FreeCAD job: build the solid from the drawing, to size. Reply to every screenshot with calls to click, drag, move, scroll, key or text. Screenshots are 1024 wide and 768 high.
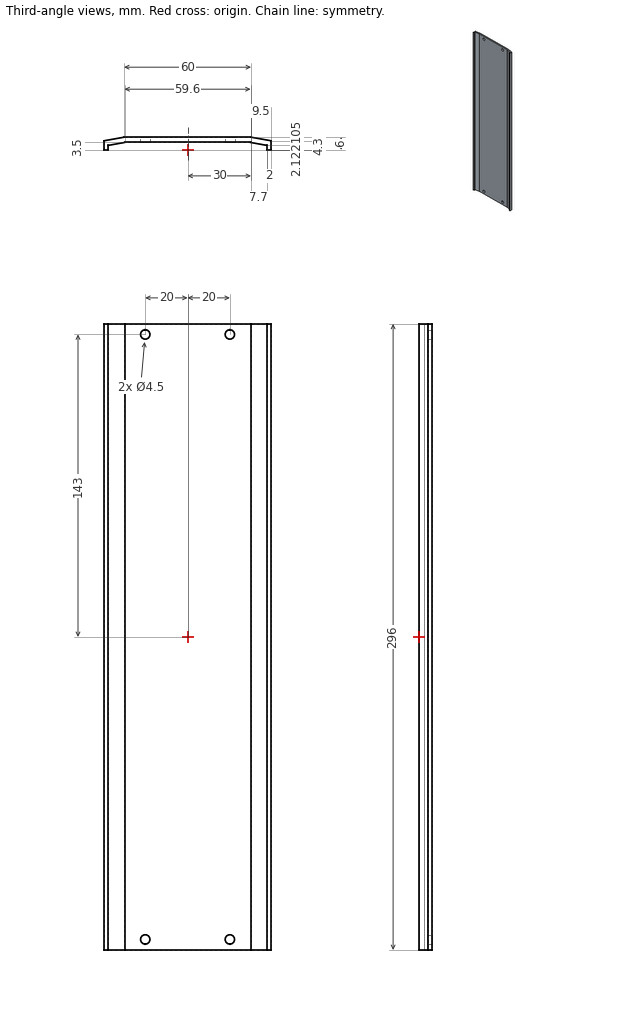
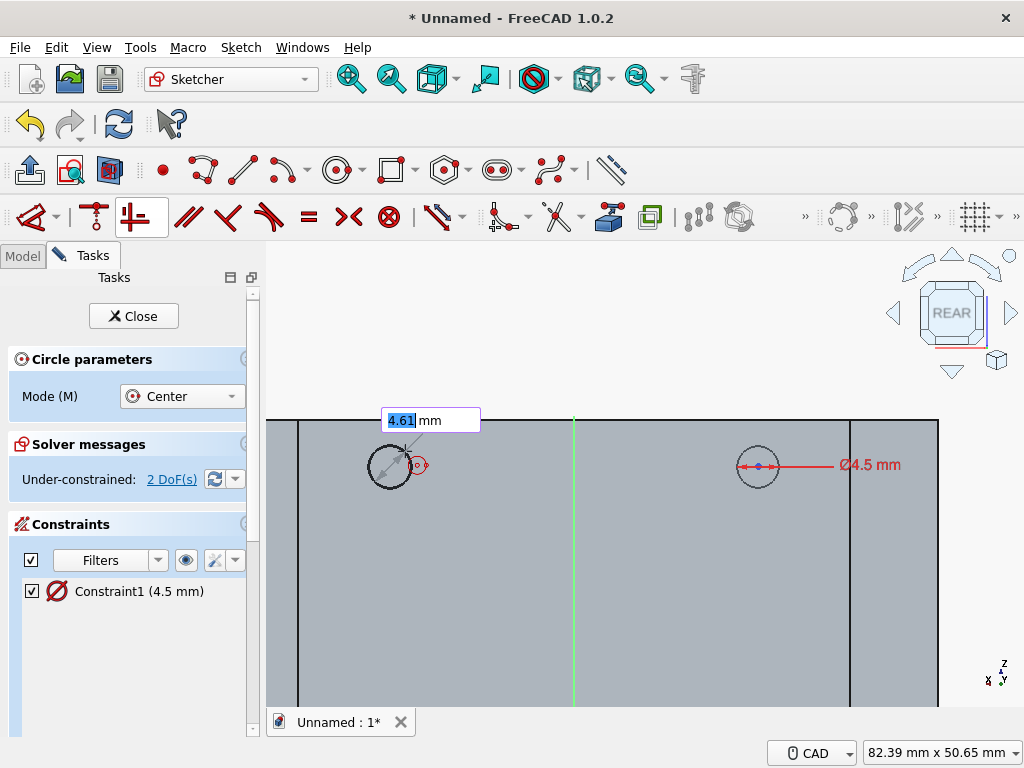
text(4.5)
key(Return)
key(Escape)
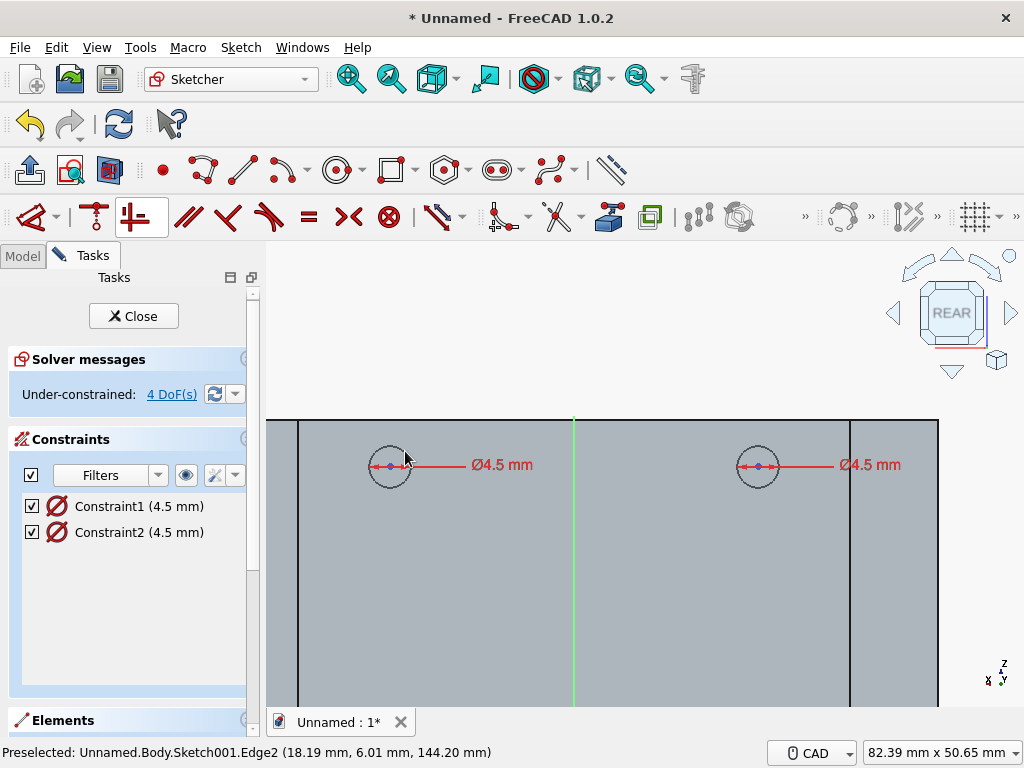
click(758, 467)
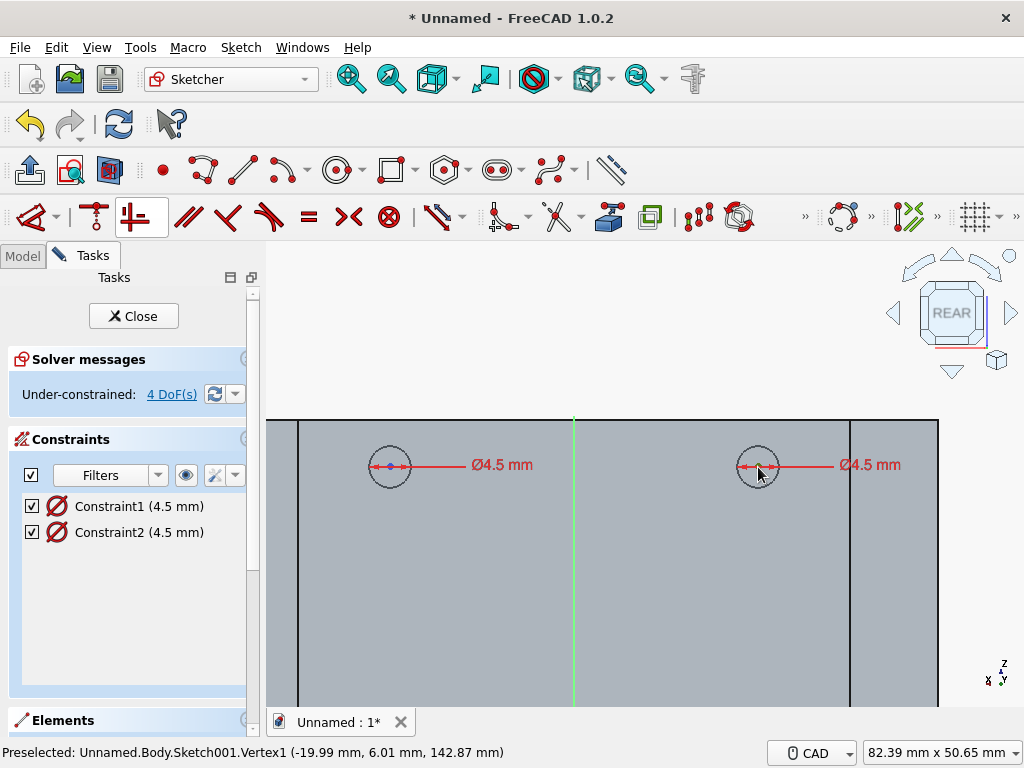
click(390, 467)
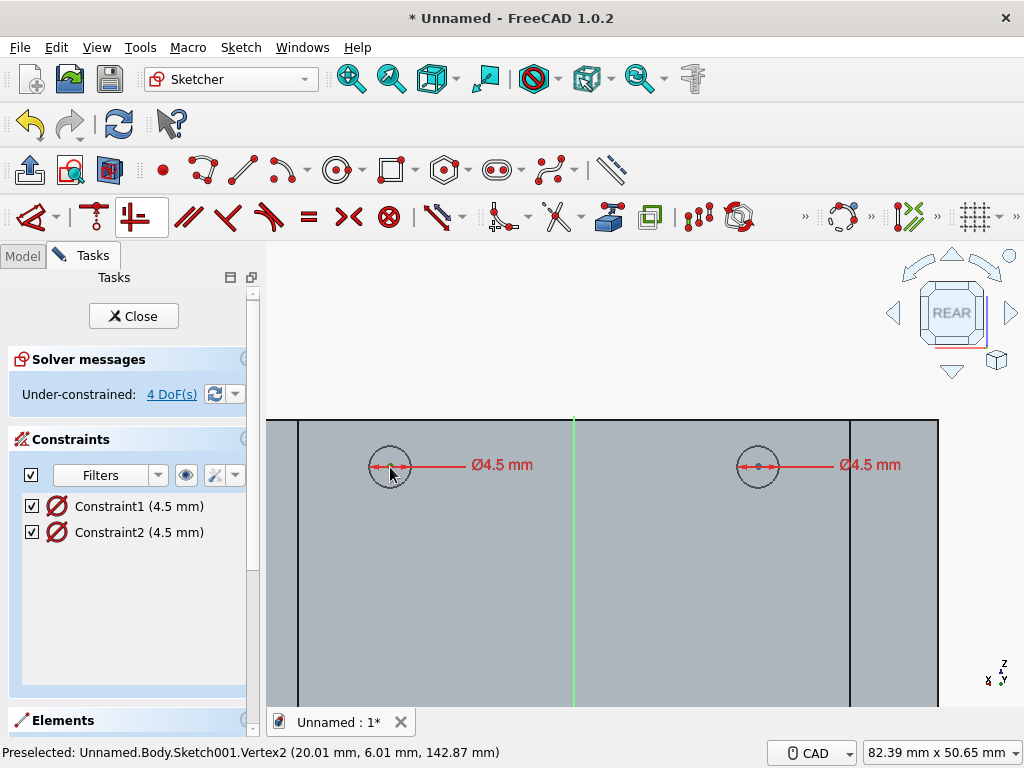
key(h)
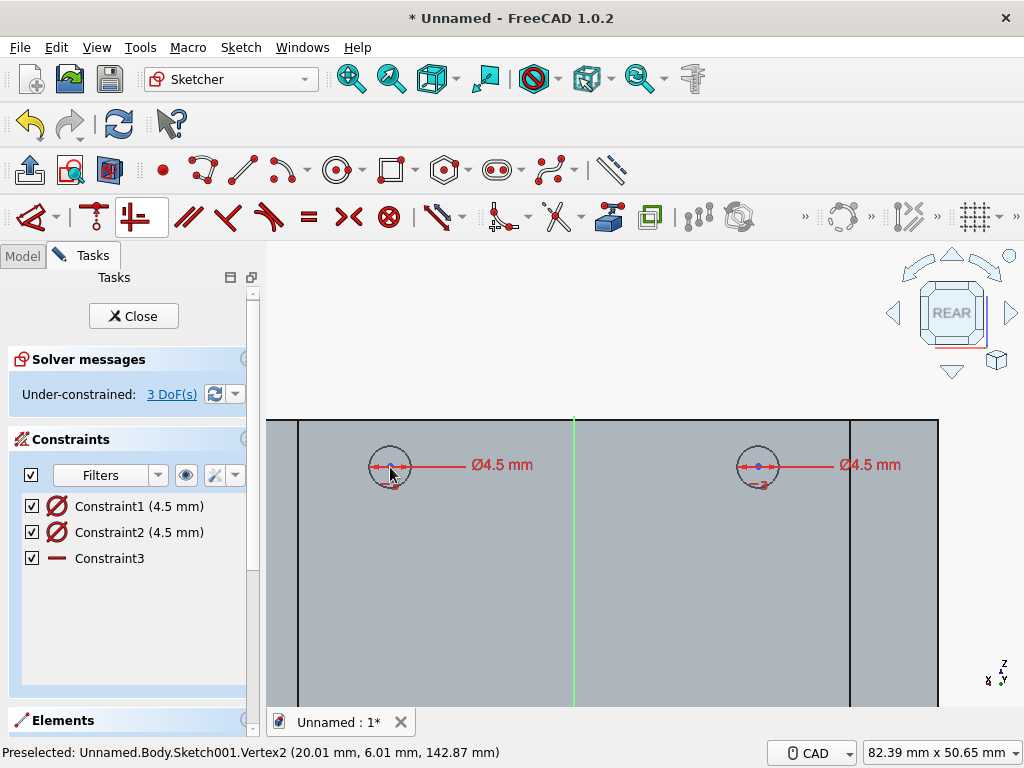
key(d)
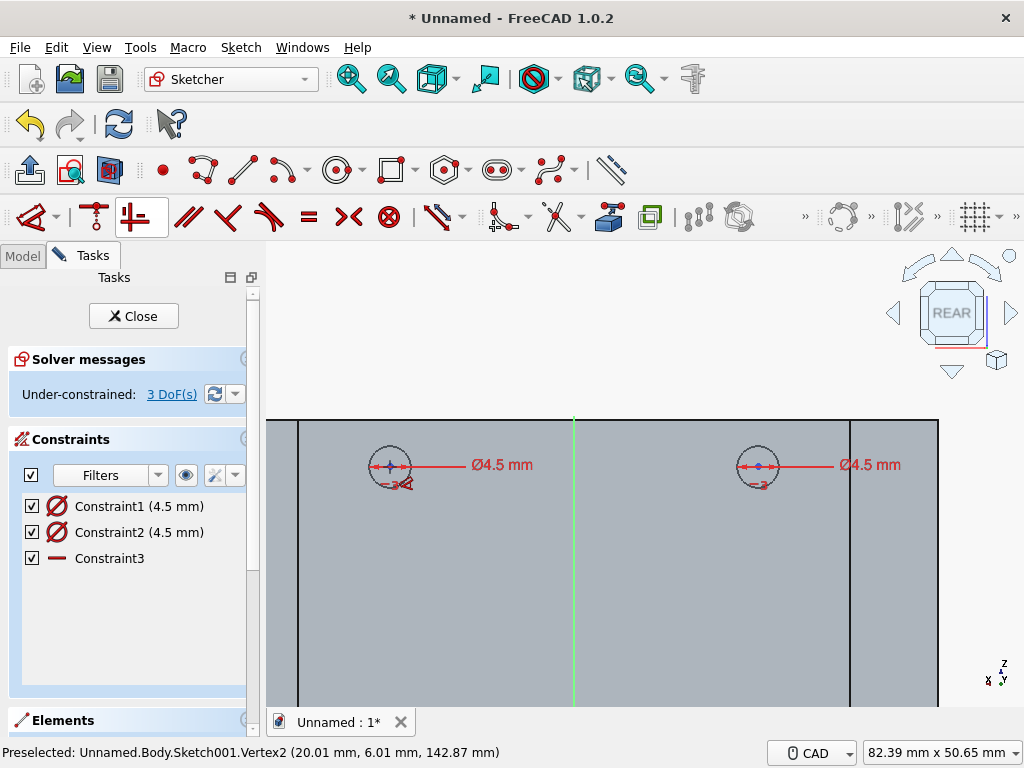
click(758, 467)
click(666, 433)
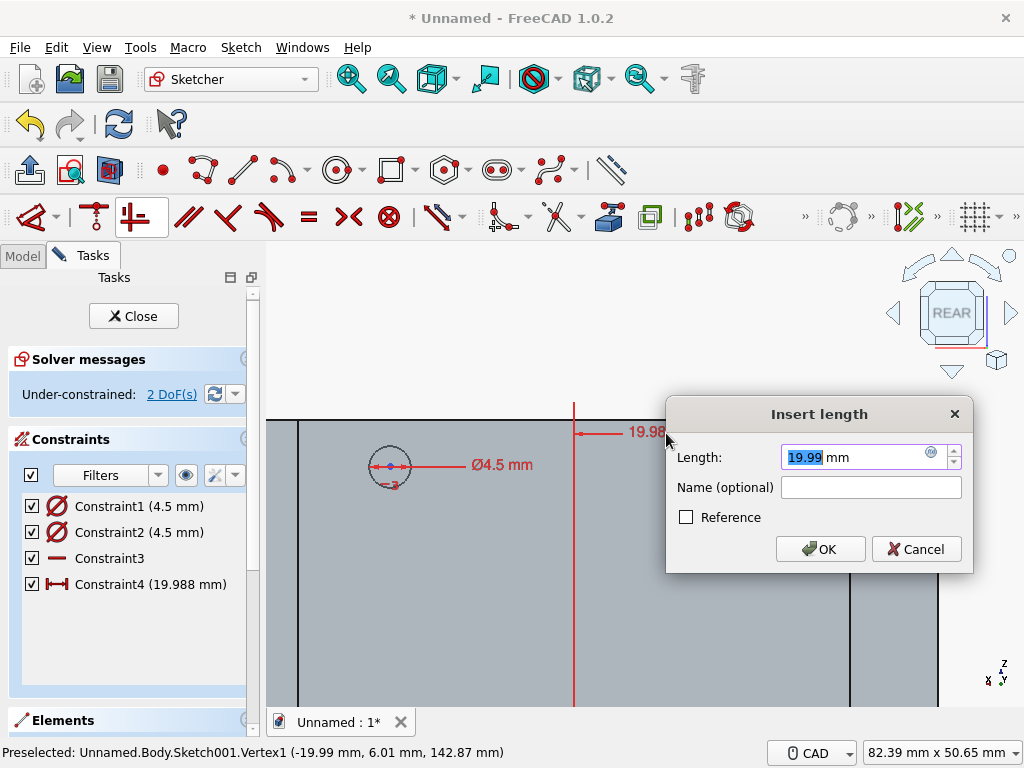
text(20)
key(Return)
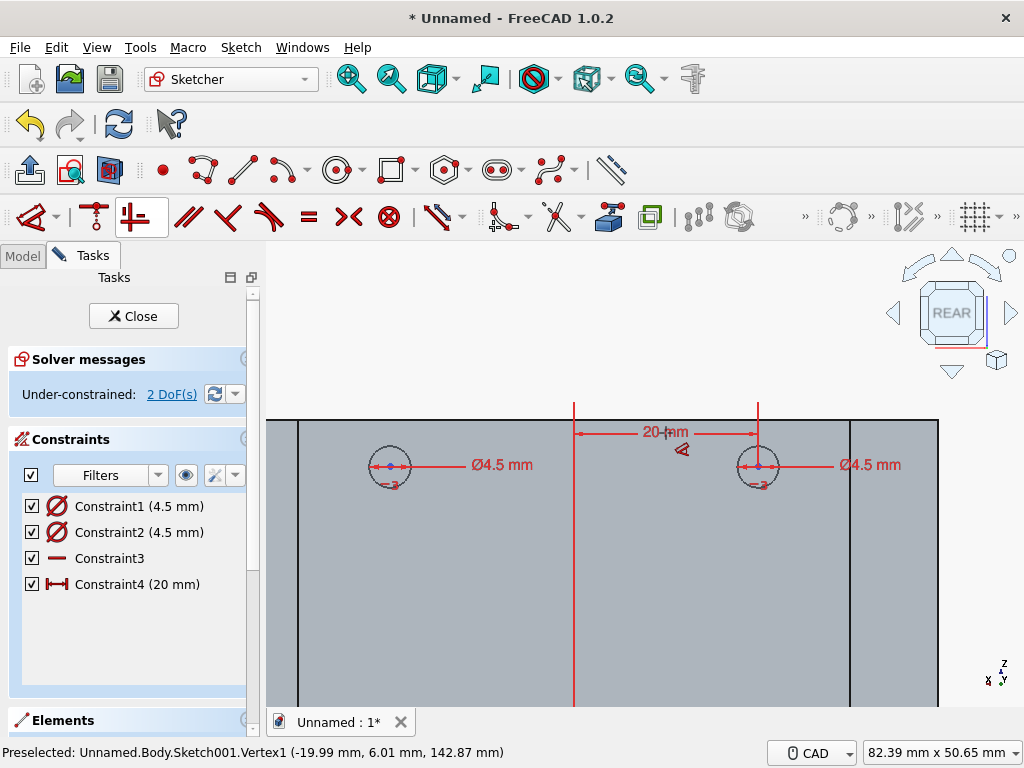
click(390, 467)
click(482, 433)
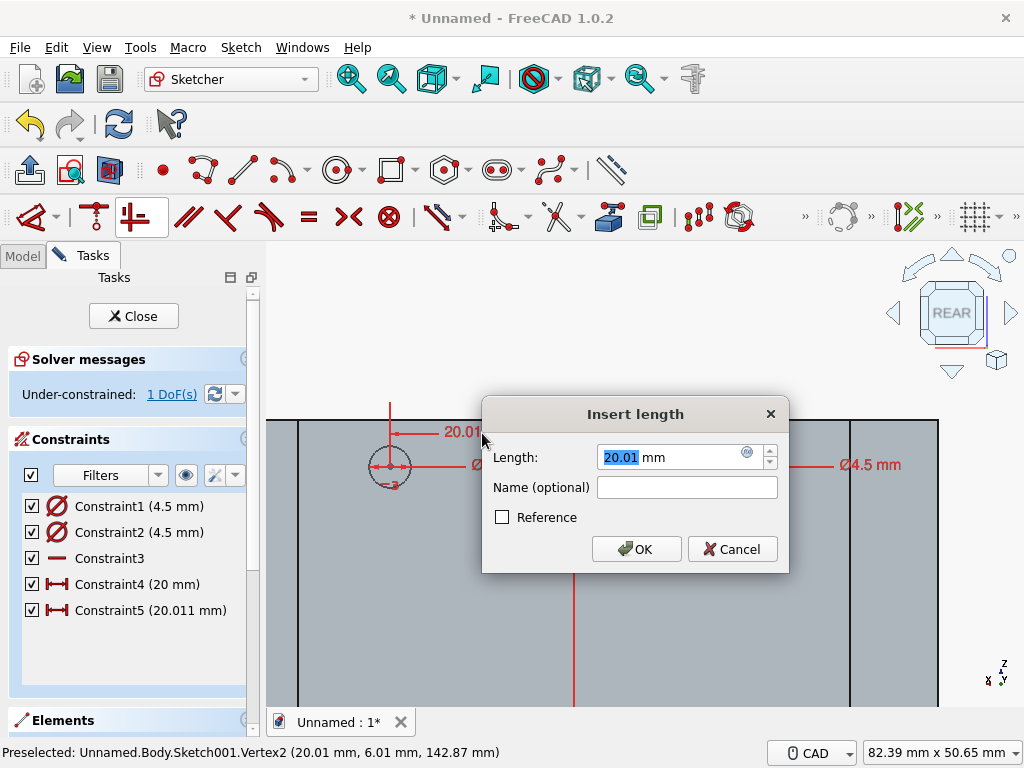
text(20)
key(Return)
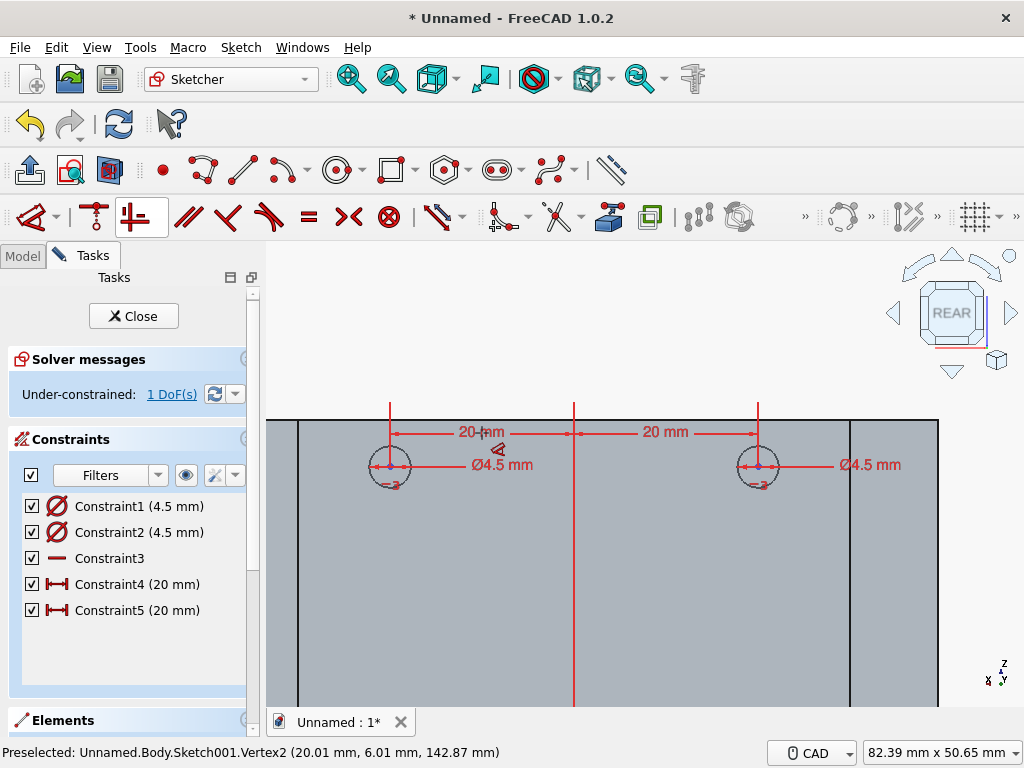
click(758, 467)
click(792, 573)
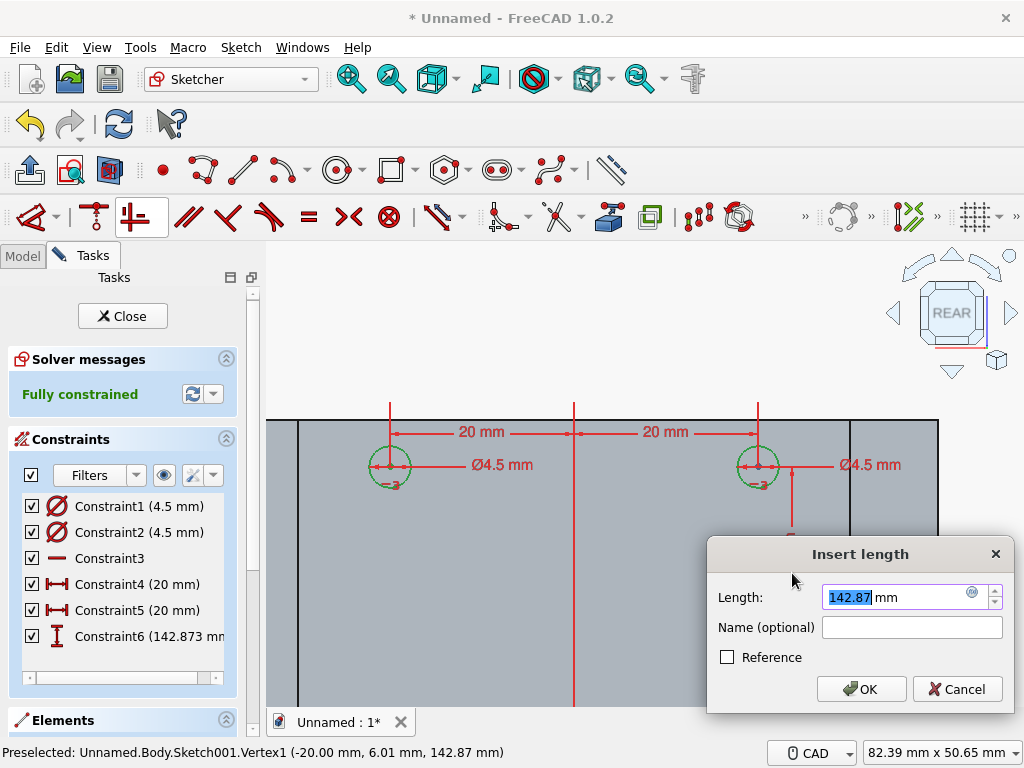
text(143)
key(Return)
key(Escape)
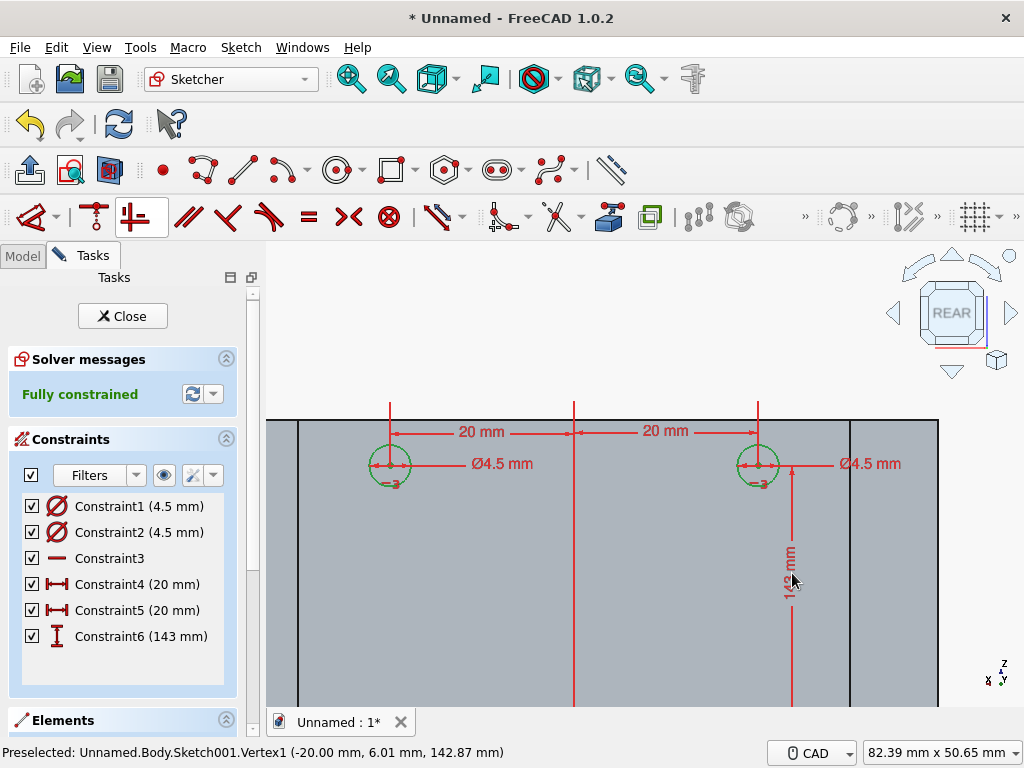
click(123, 316)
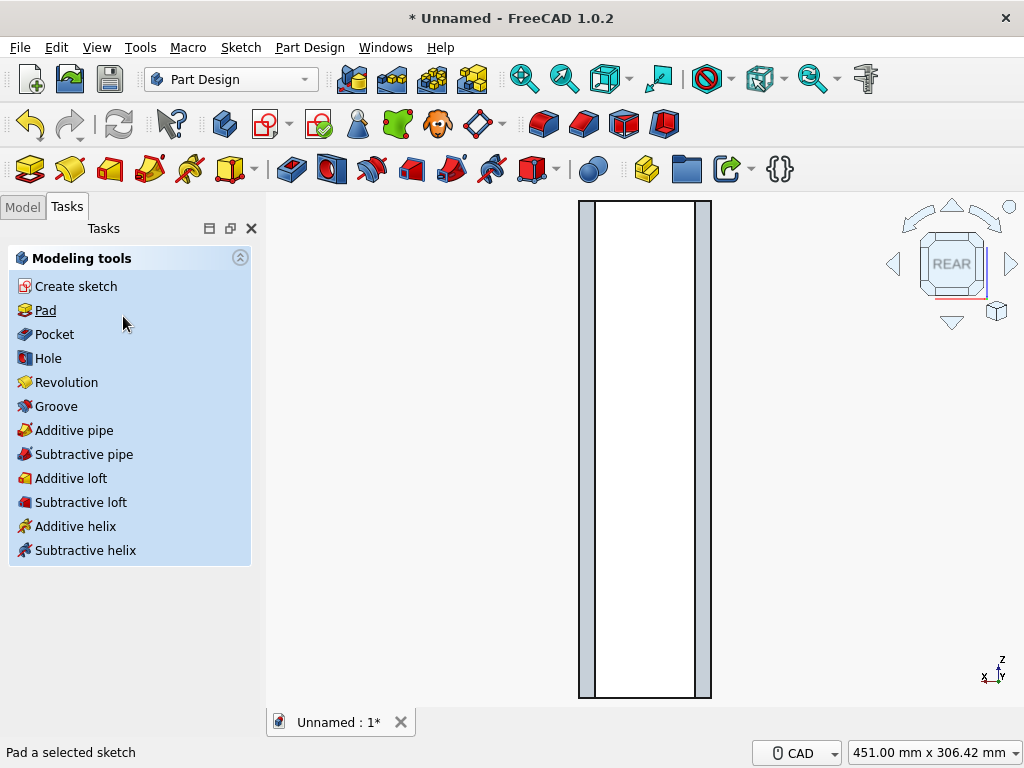
click(292, 170)